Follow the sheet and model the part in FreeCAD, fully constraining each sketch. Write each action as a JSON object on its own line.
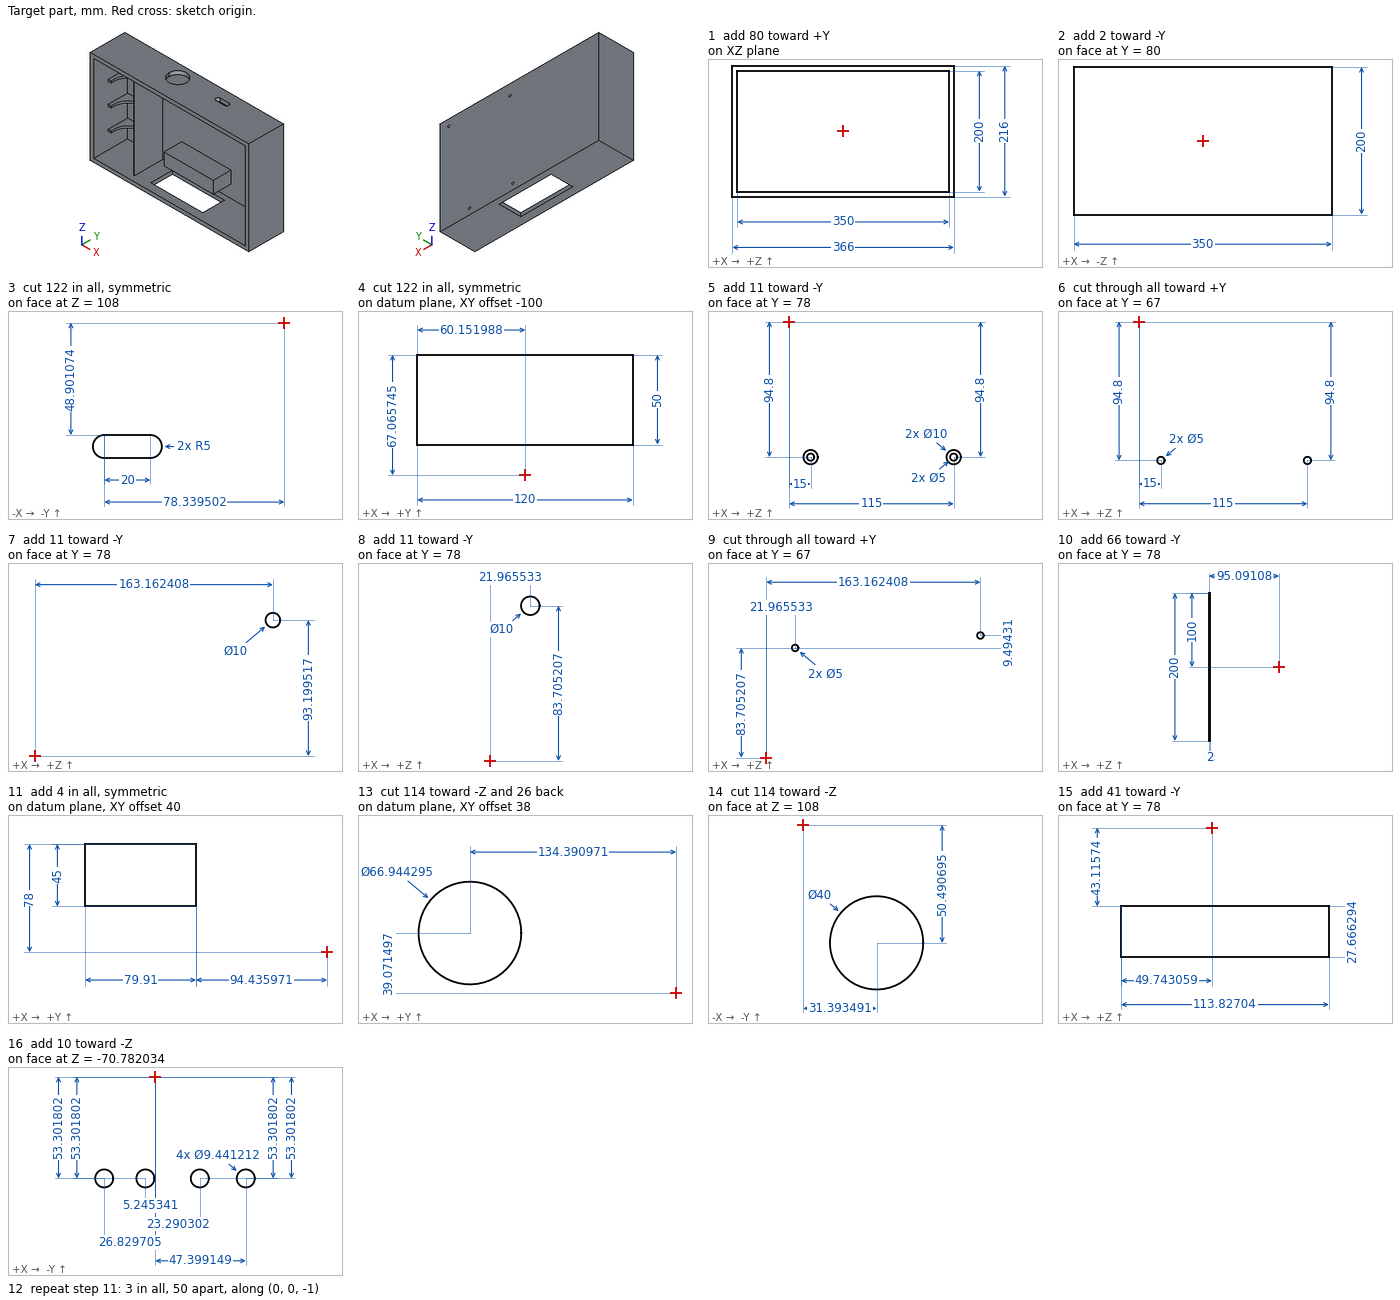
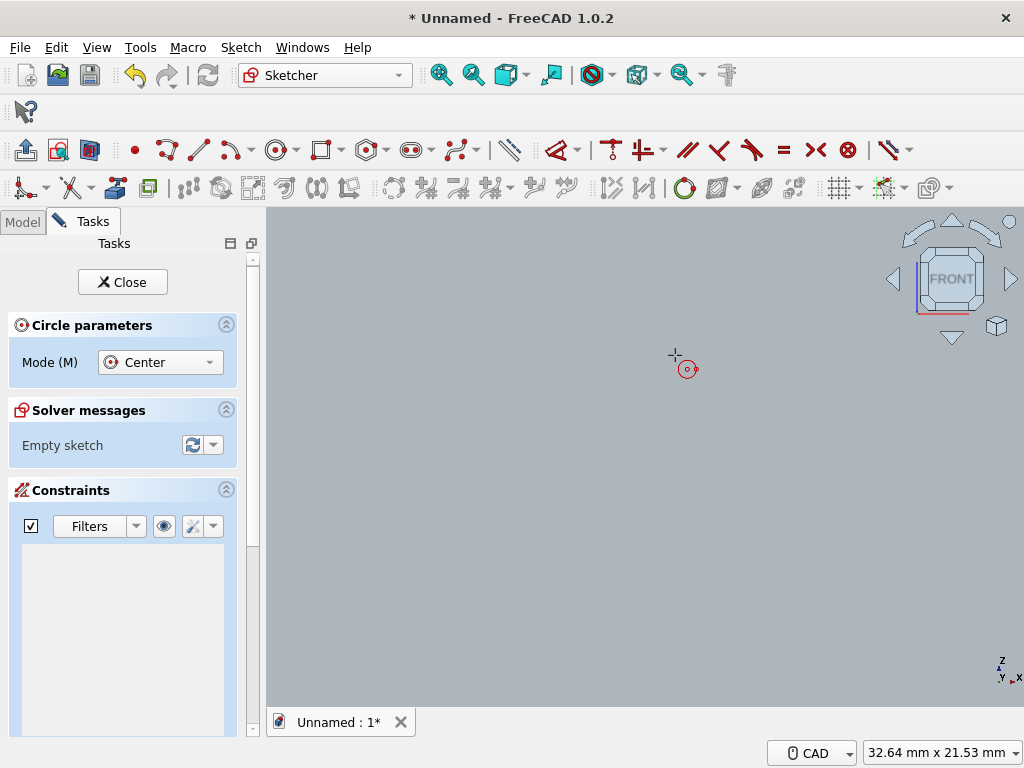
{"action": "left_click", "coordinate": [572, 454]}
{"action": "mouse_move", "coordinate": [654, 372]}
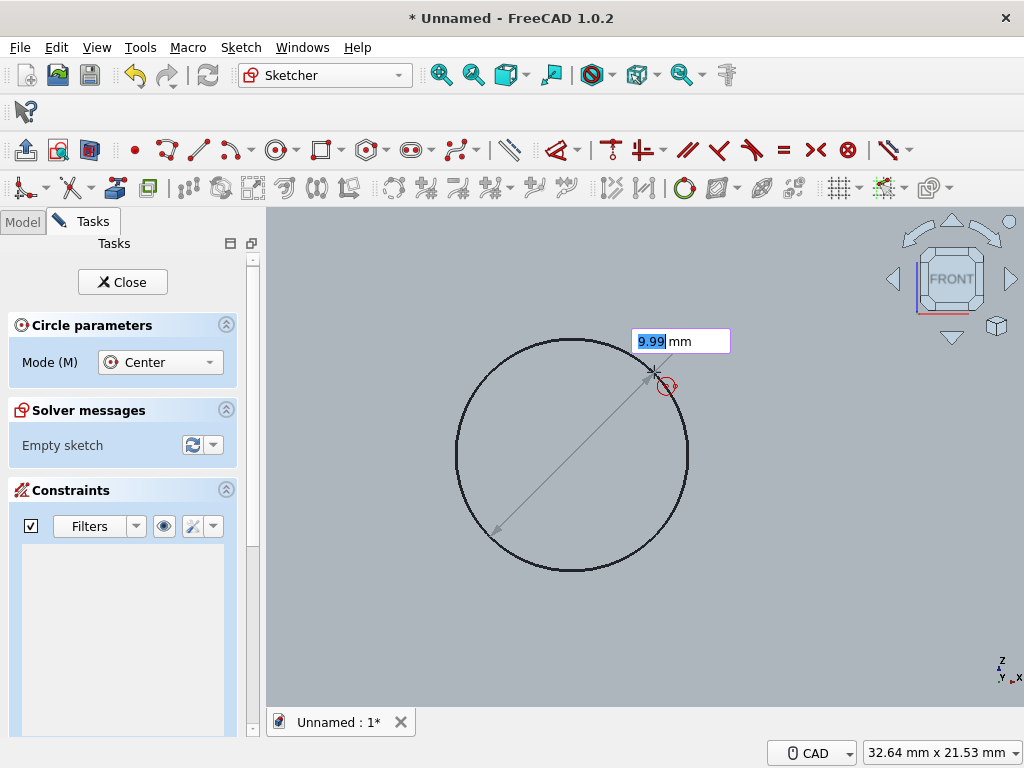
{"action": "type", "text": "10"}
{"action": "key", "text": "Return"}
{"action": "key", "text": "Escape"}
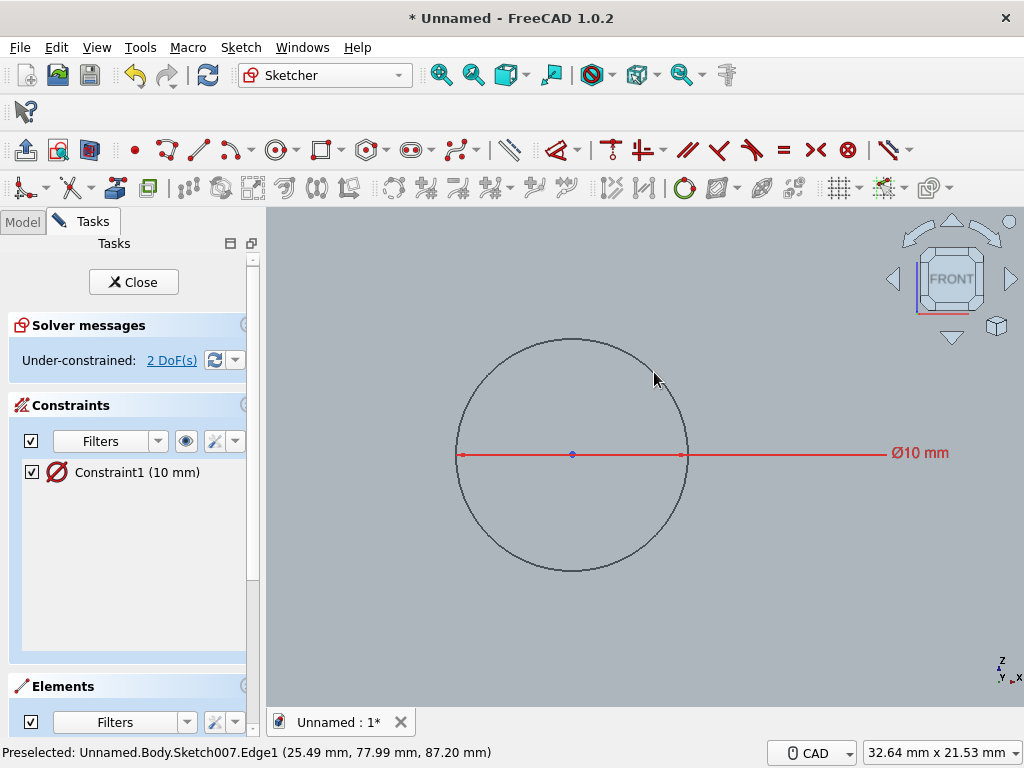
{"action": "key", "text": "d"}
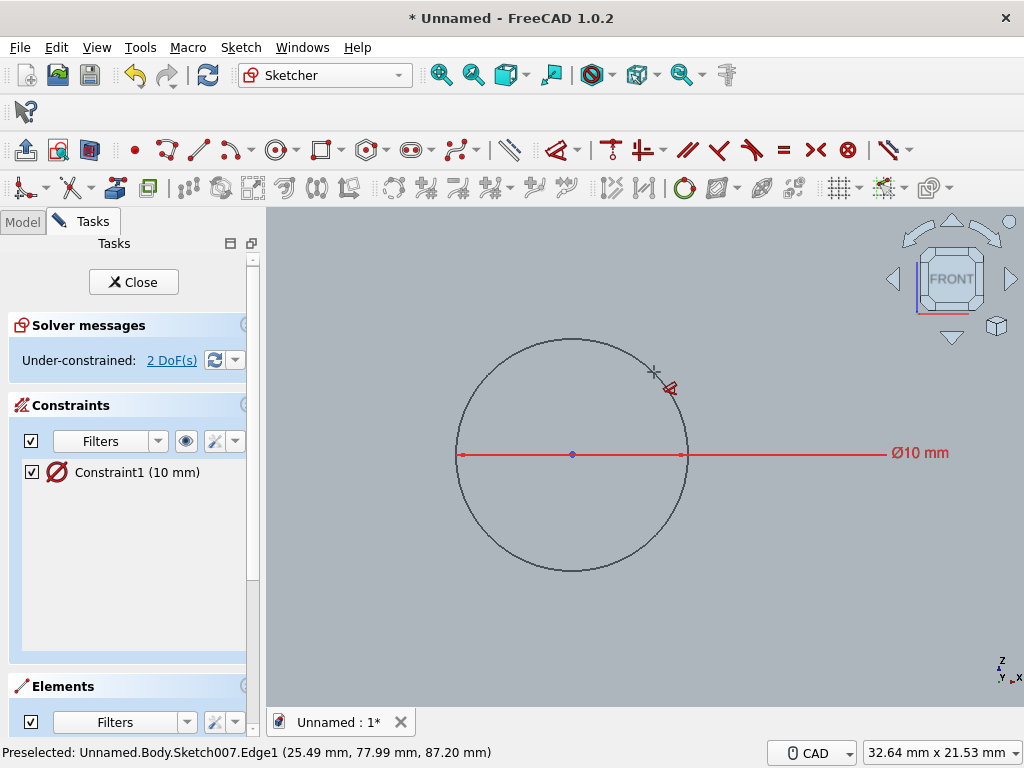
{"action": "left_click", "coordinate": [572, 455]}
{"action": "left_click", "coordinate": [433, 421]}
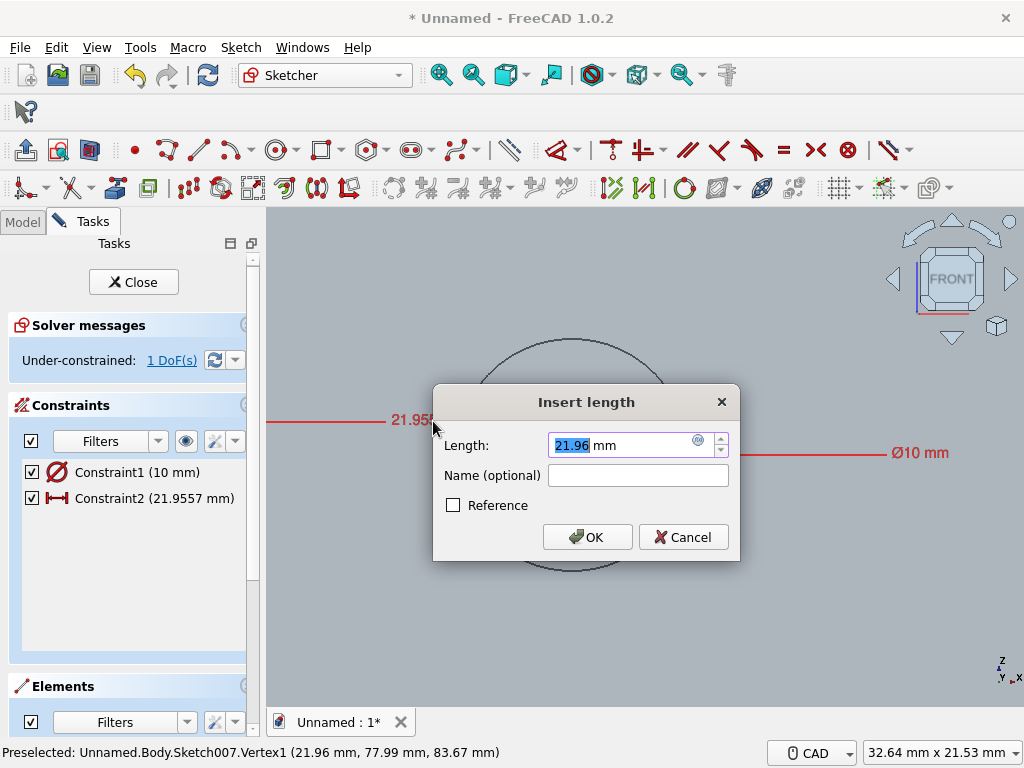
{"action": "type", "text": "21.965533"}
{"action": "key", "text": "Return"}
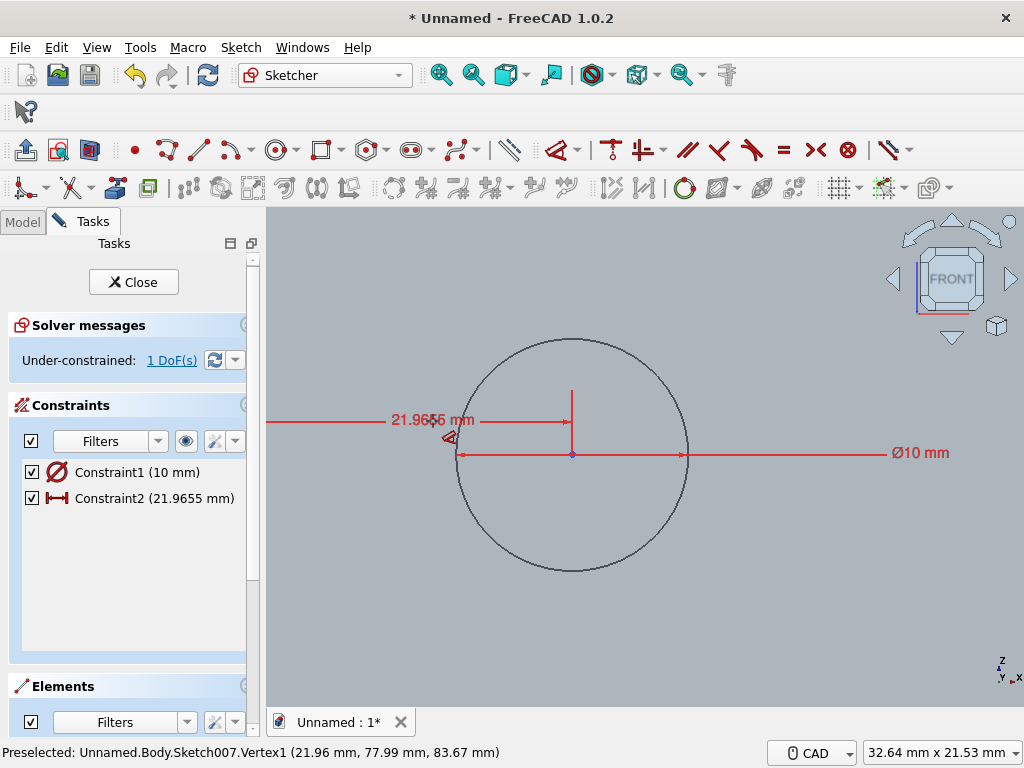
{"action": "left_click", "coordinate": [572, 455]}
{"action": "left_click", "coordinate": [606, 515]}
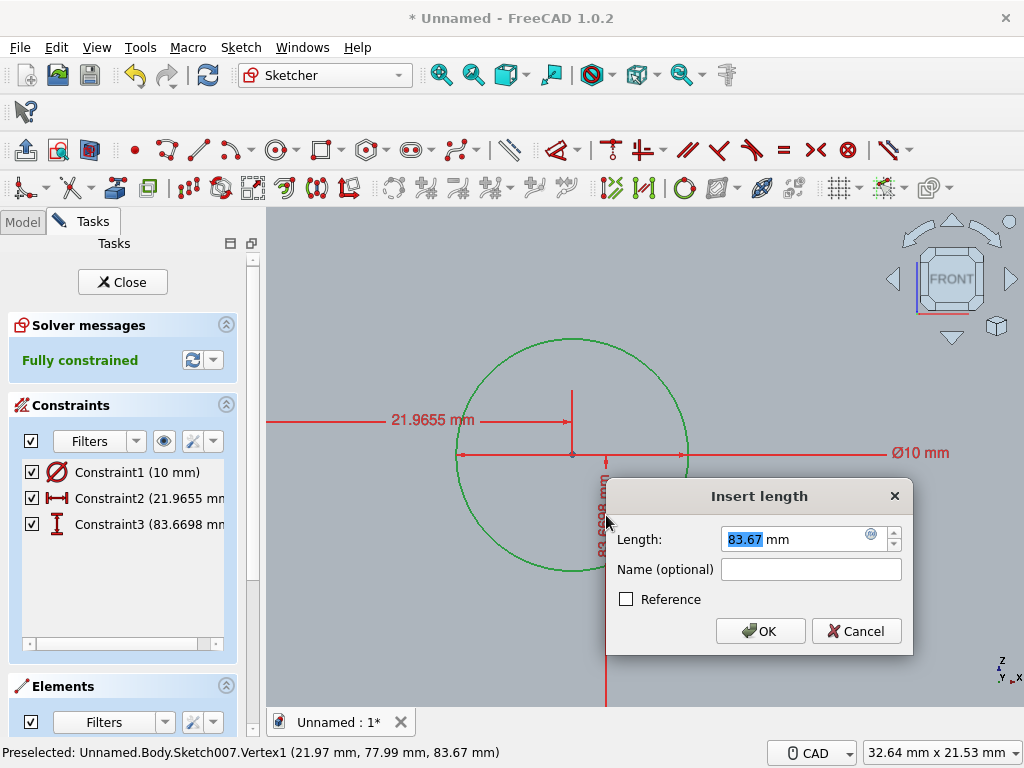
{"action": "type", "text": "83.705207"}
{"action": "key", "text": "Return"}
{"action": "key", "text": "Escape"}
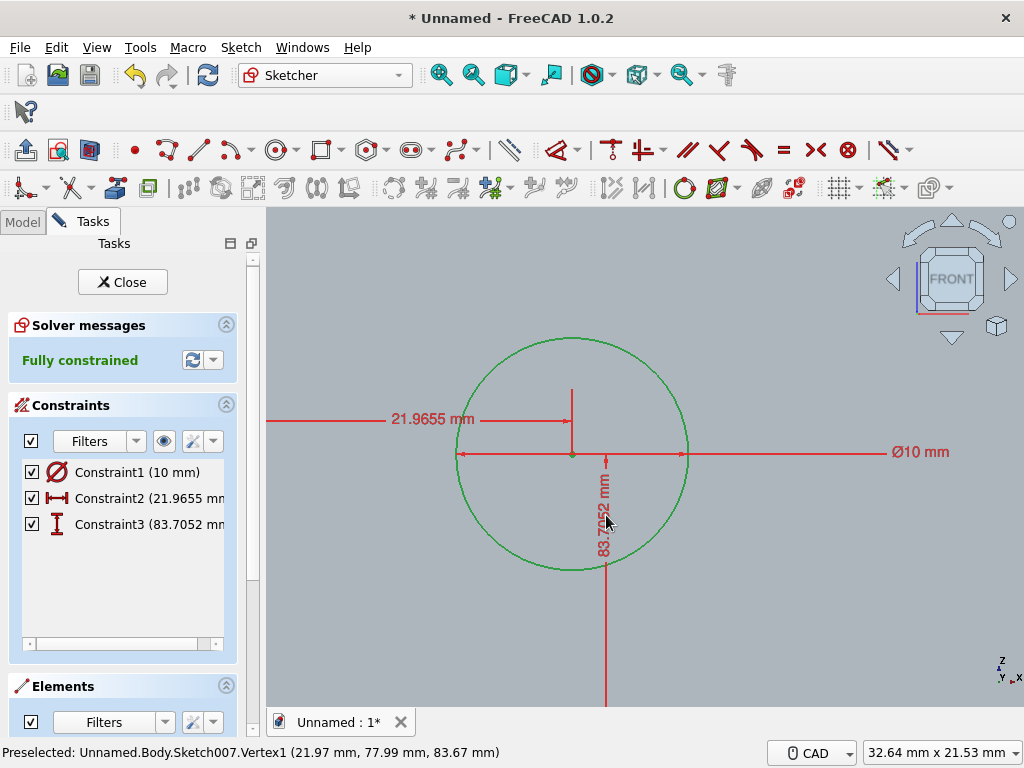
{"action": "left_click", "coordinate": [123, 282]}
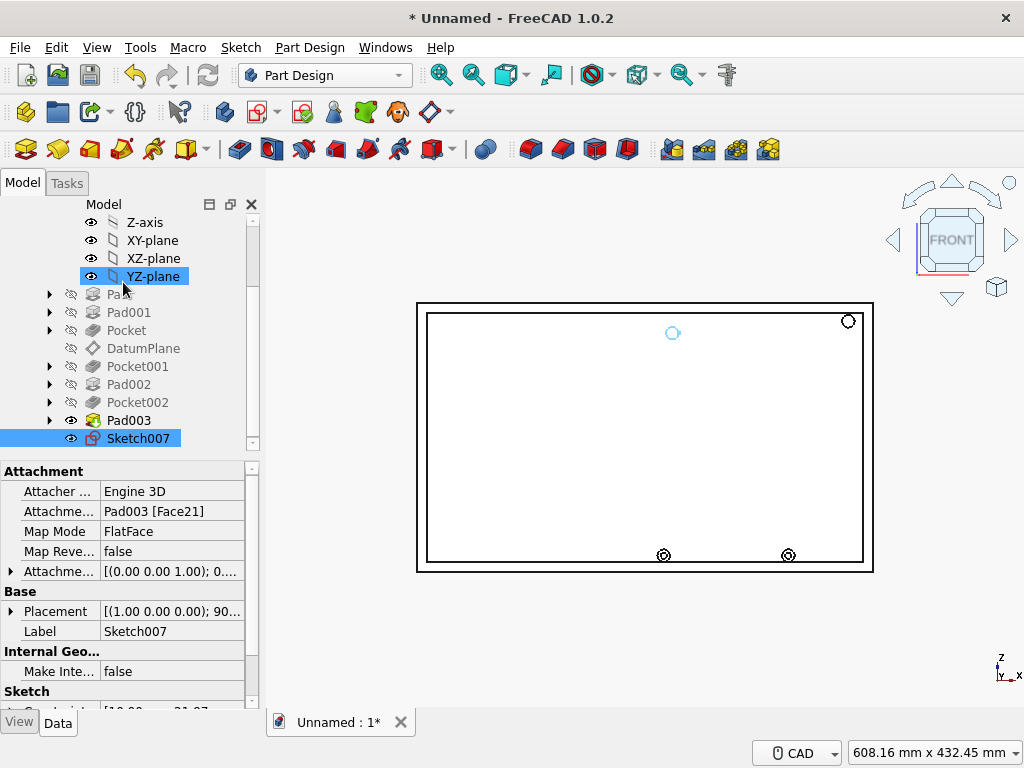
{"action": "left_click", "coordinate": [26, 150]}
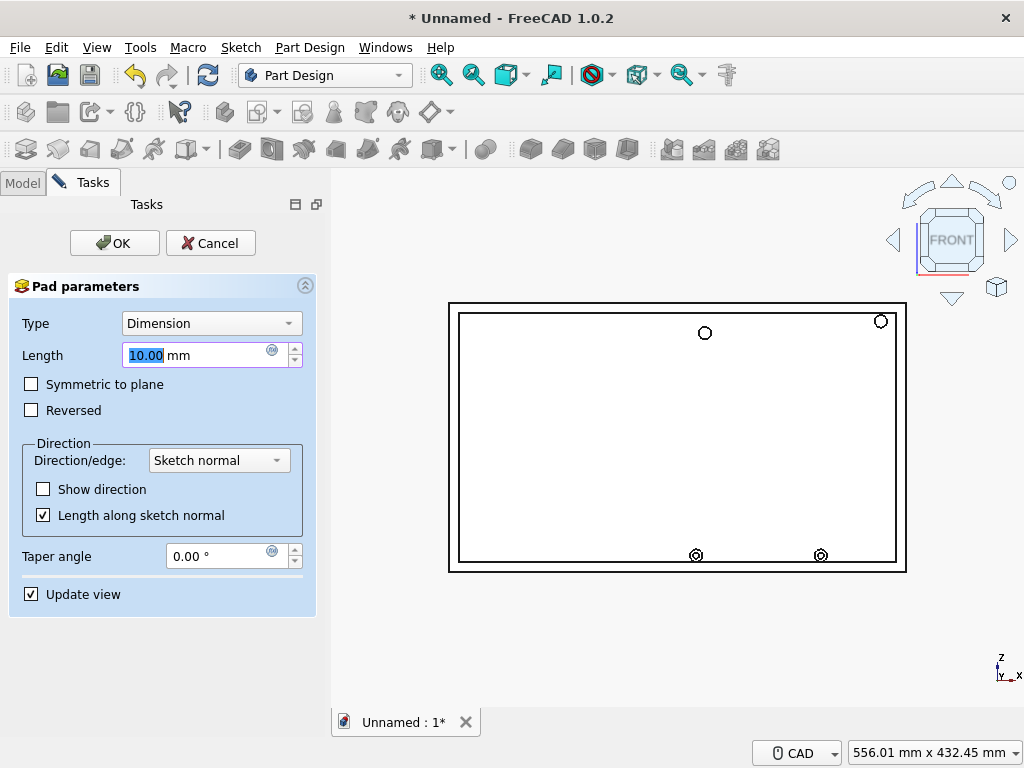
{"action": "type", "text": "11"}
{"action": "key", "text": "Tab"}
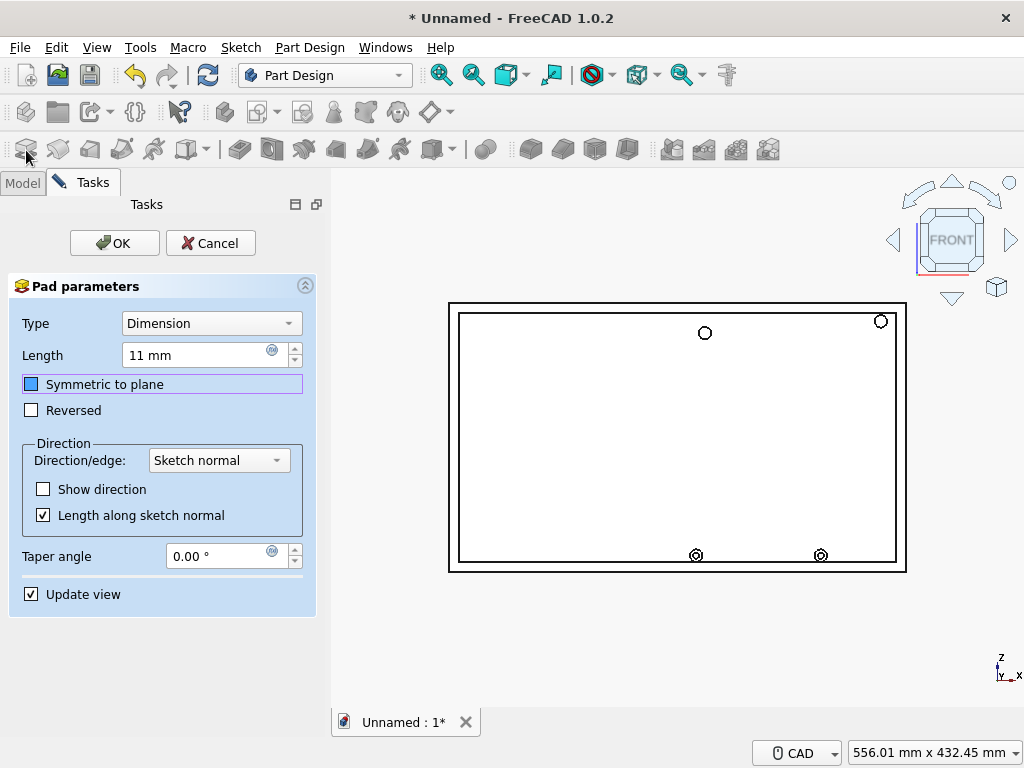
{"action": "left_click", "coordinate": [115, 243]}